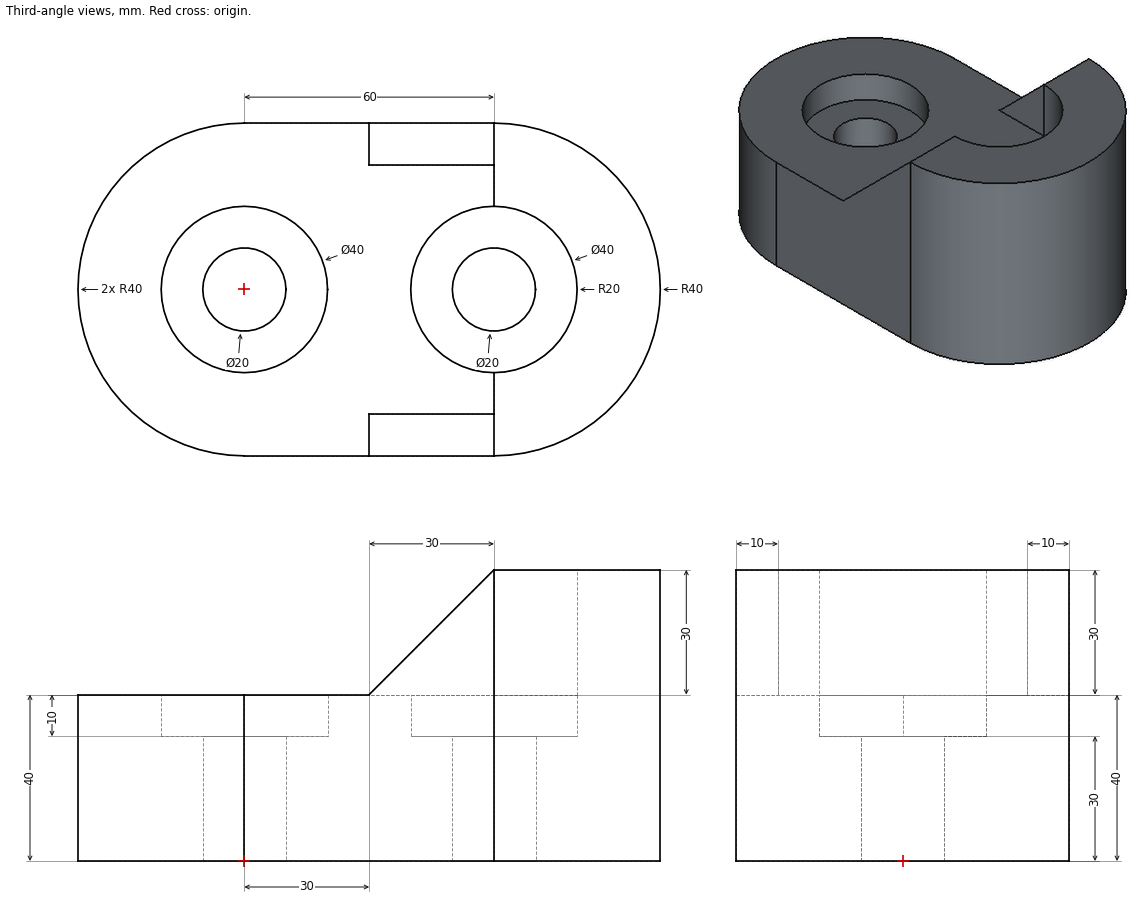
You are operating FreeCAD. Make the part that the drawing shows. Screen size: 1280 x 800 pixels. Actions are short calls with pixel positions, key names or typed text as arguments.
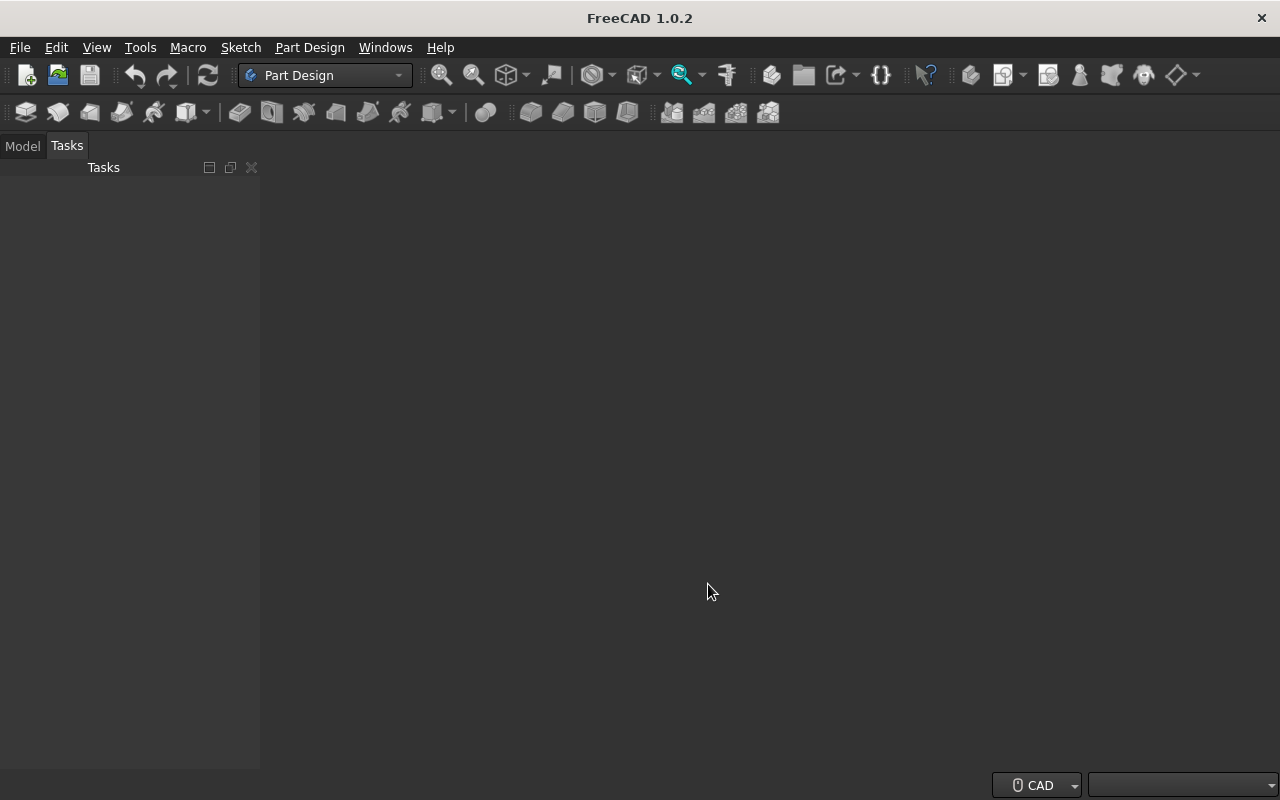
click(26, 76)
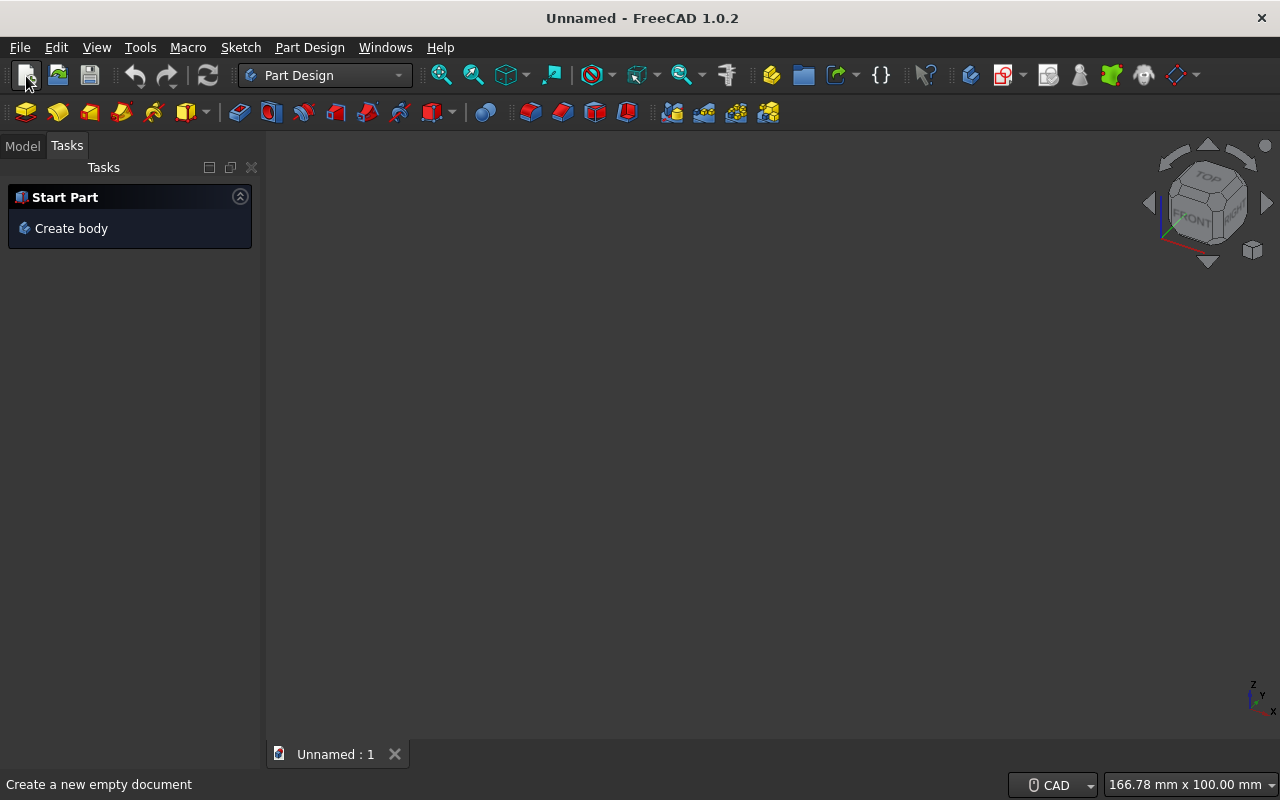
click(1004, 76)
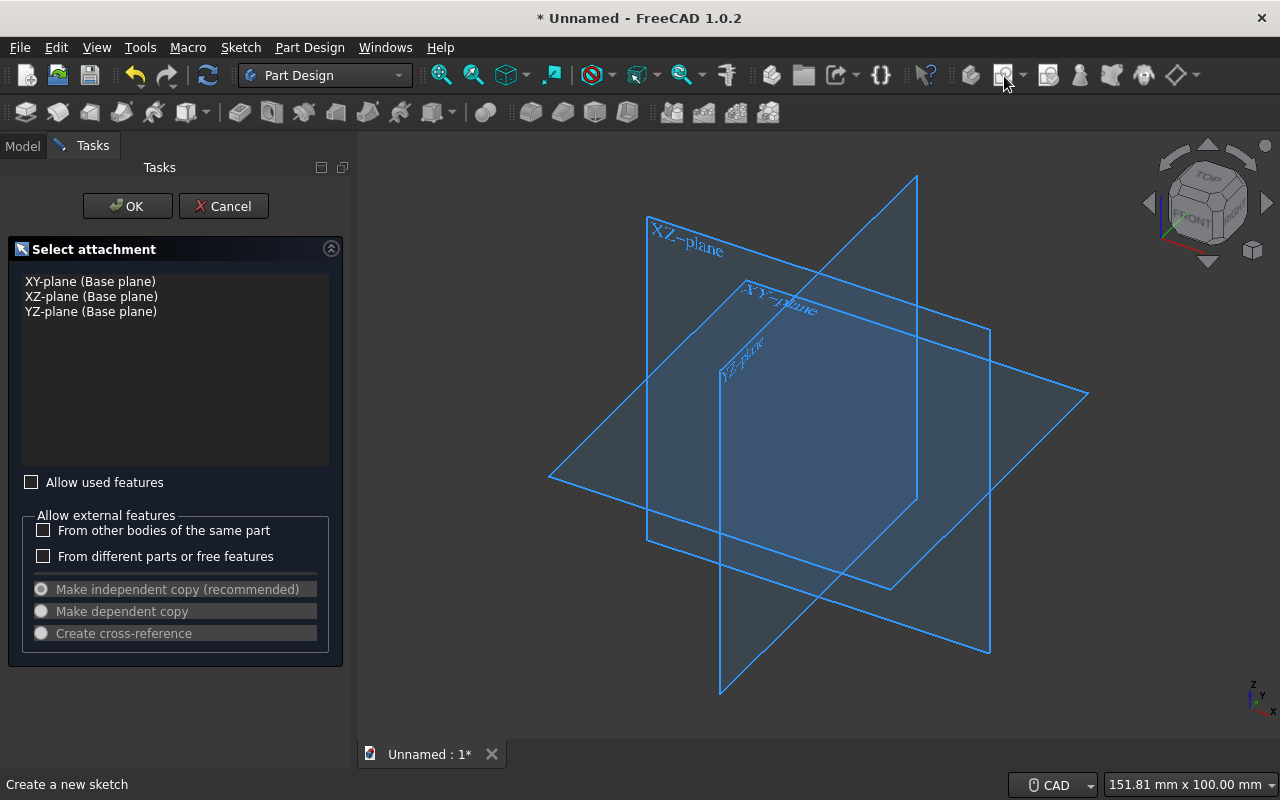
click(82, 282)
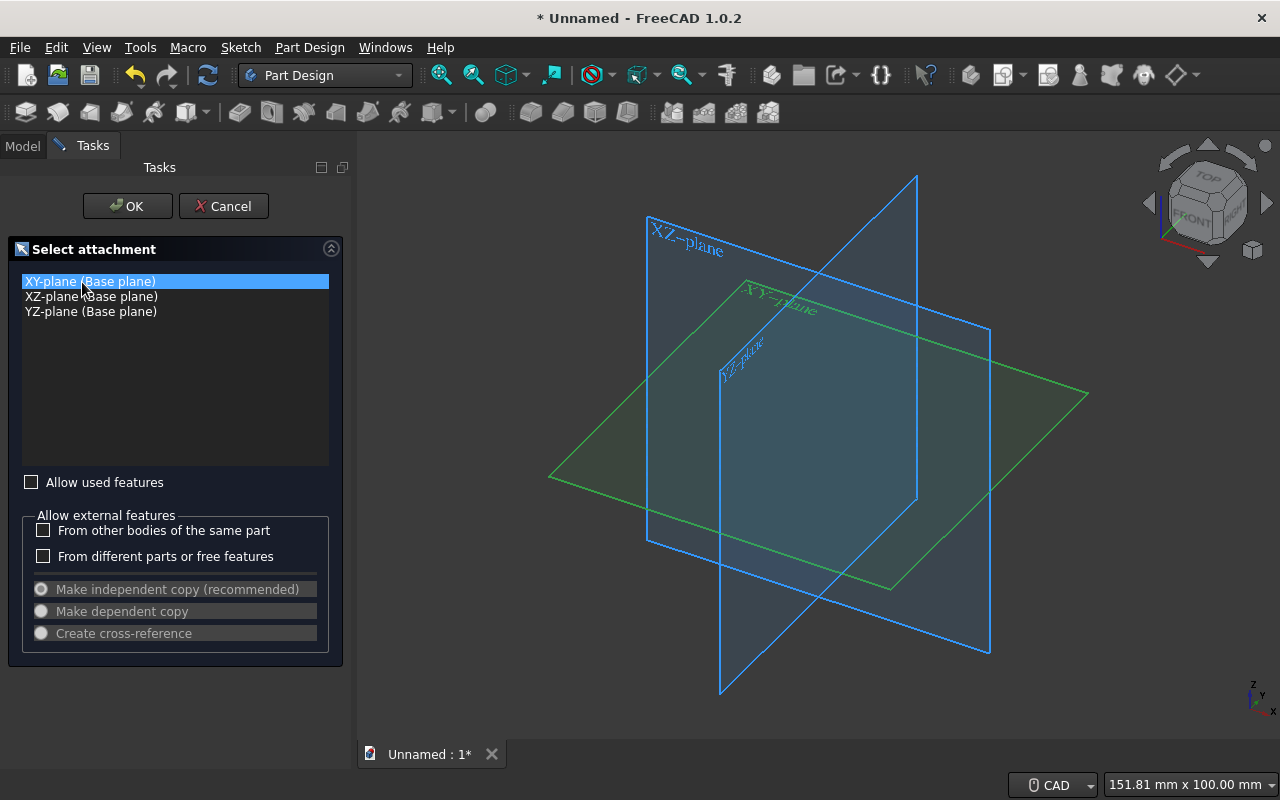
click(128, 206)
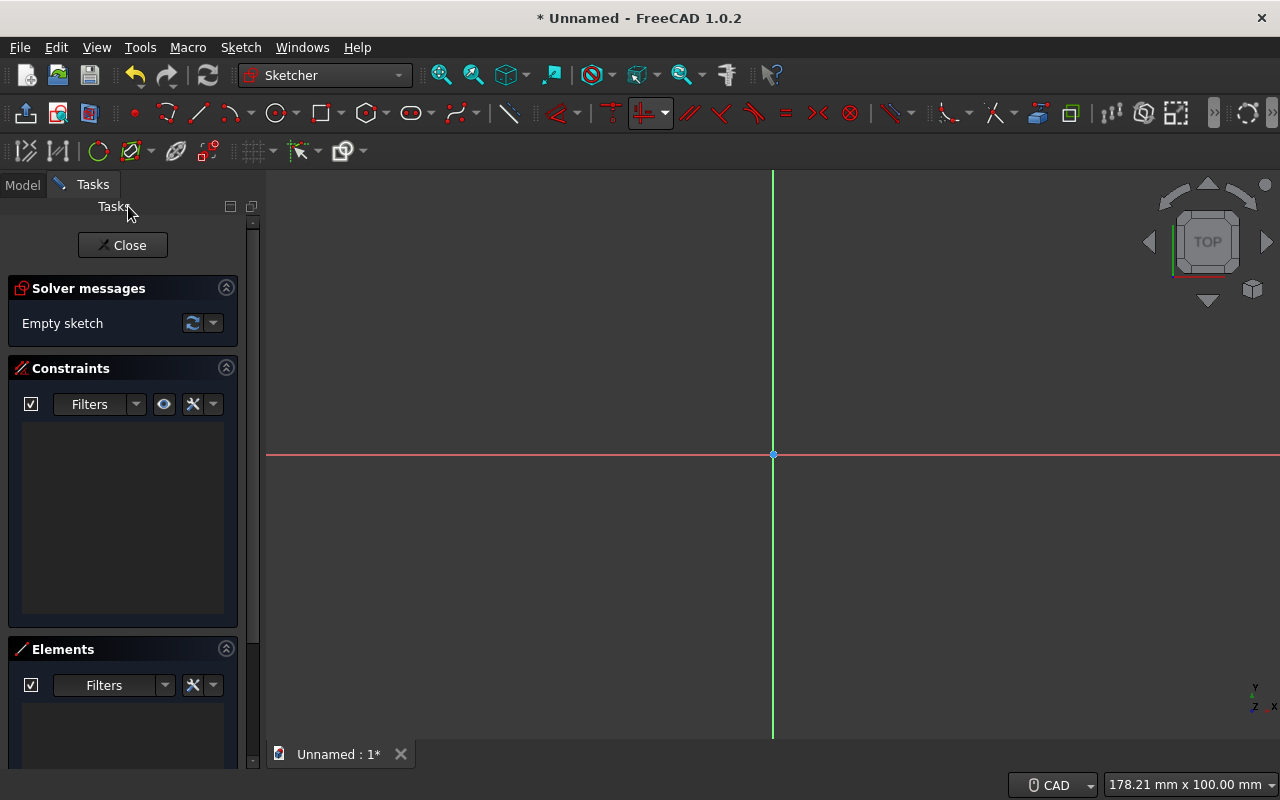
scroll(294, 455, down, 2)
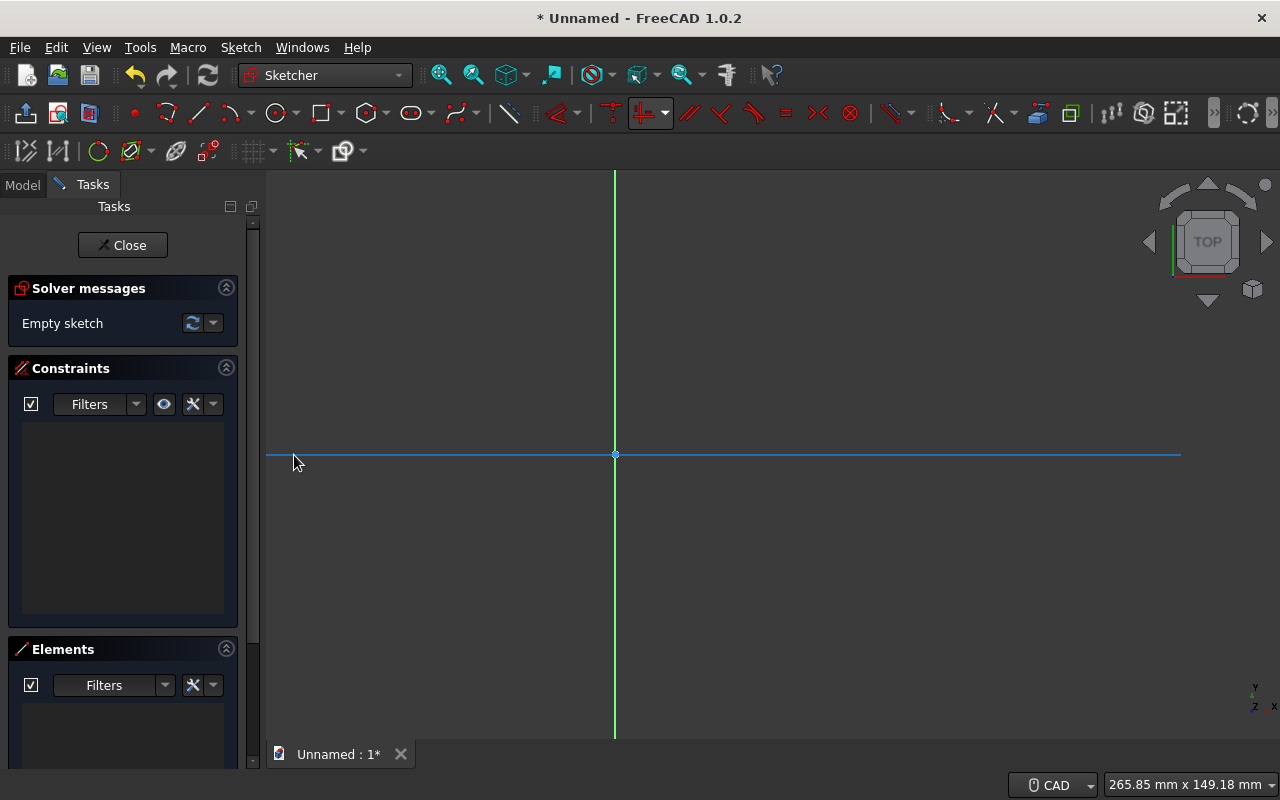
click(412, 114)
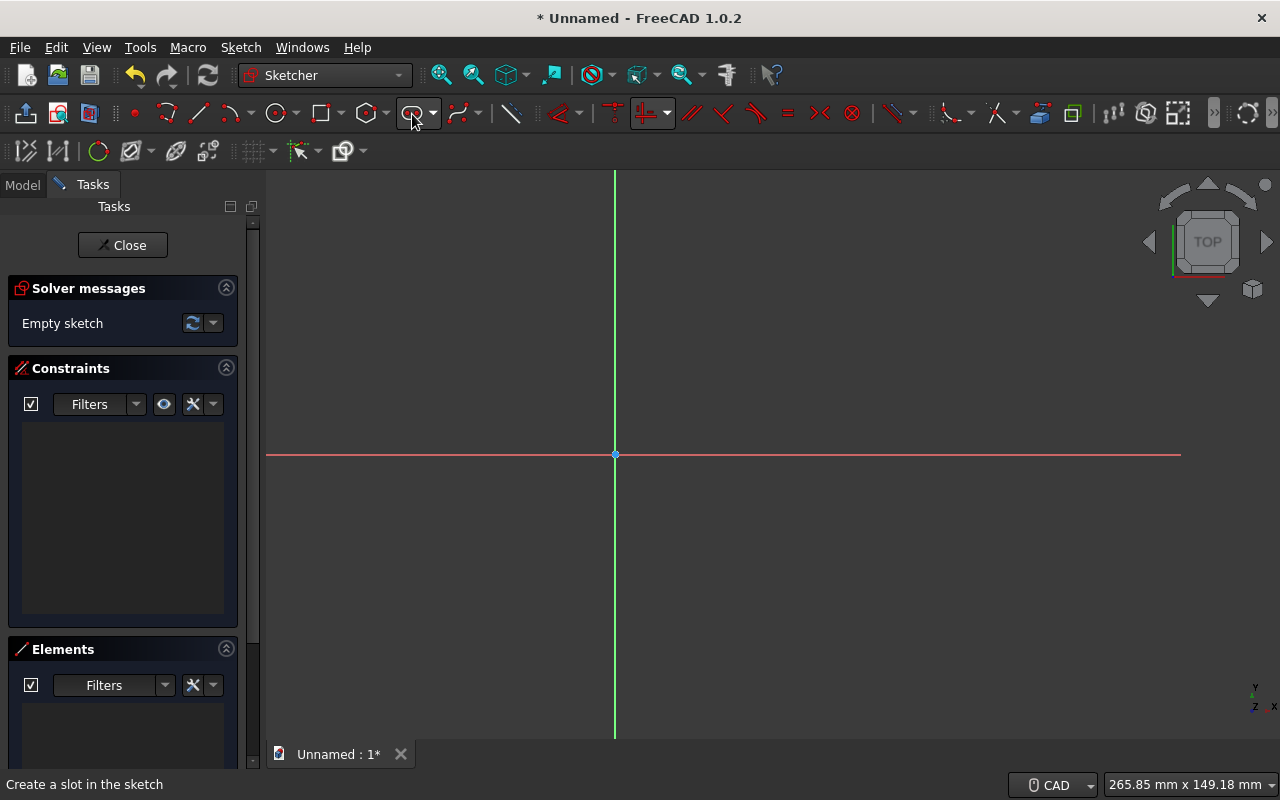
click(615, 455)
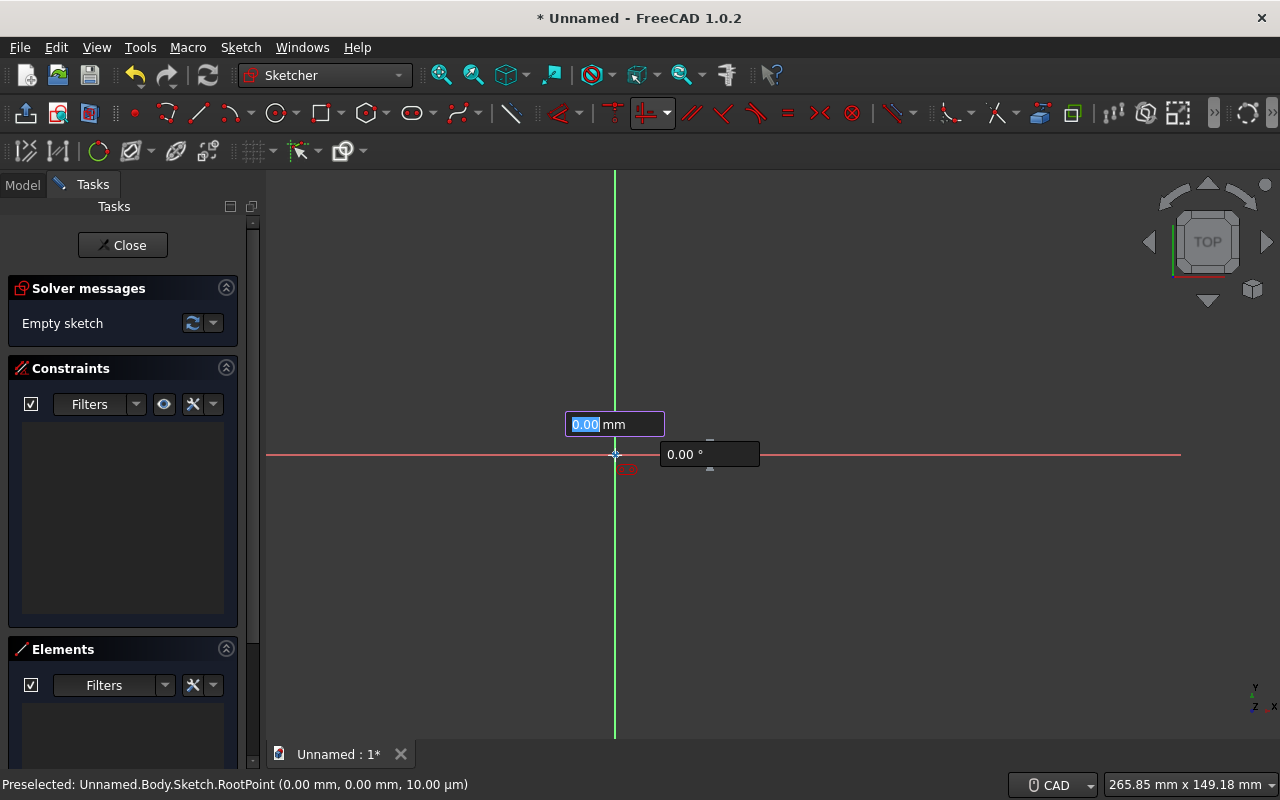
click(844, 446)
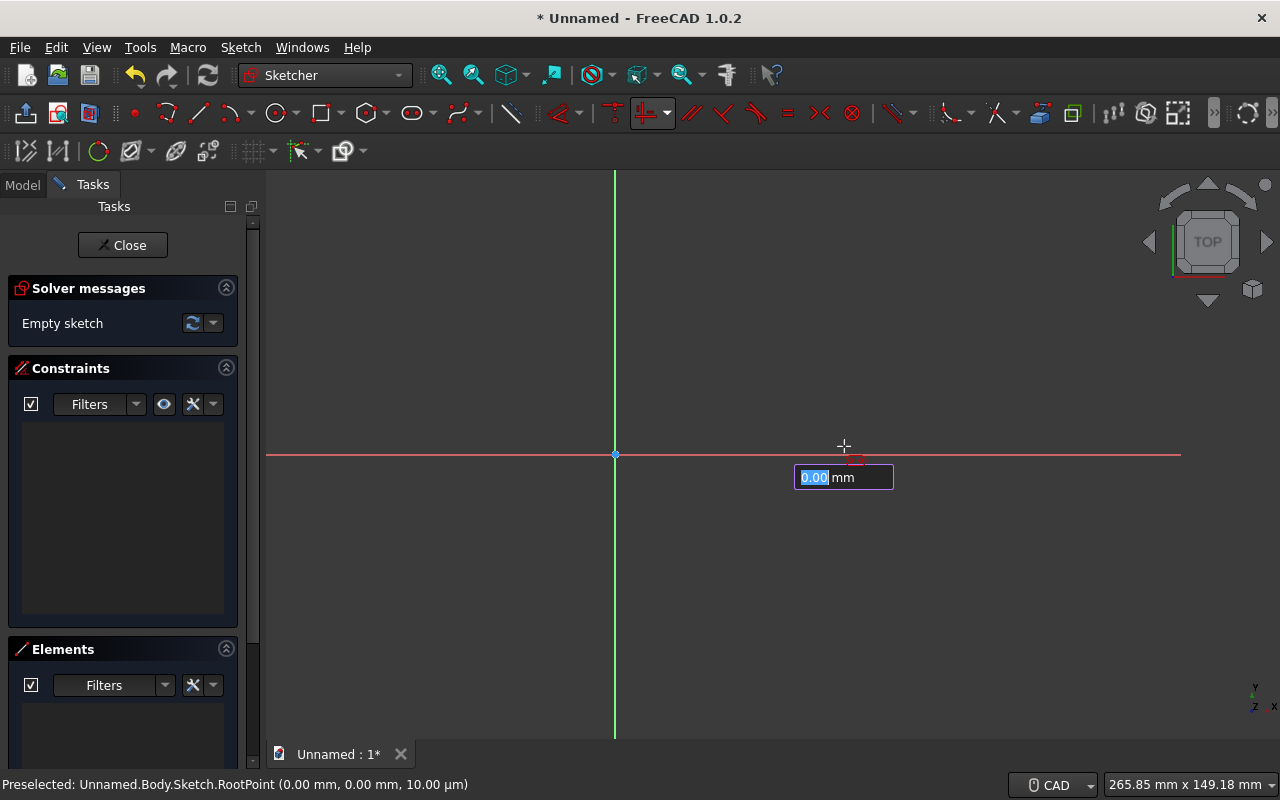
click(730, 302)
key(Escape)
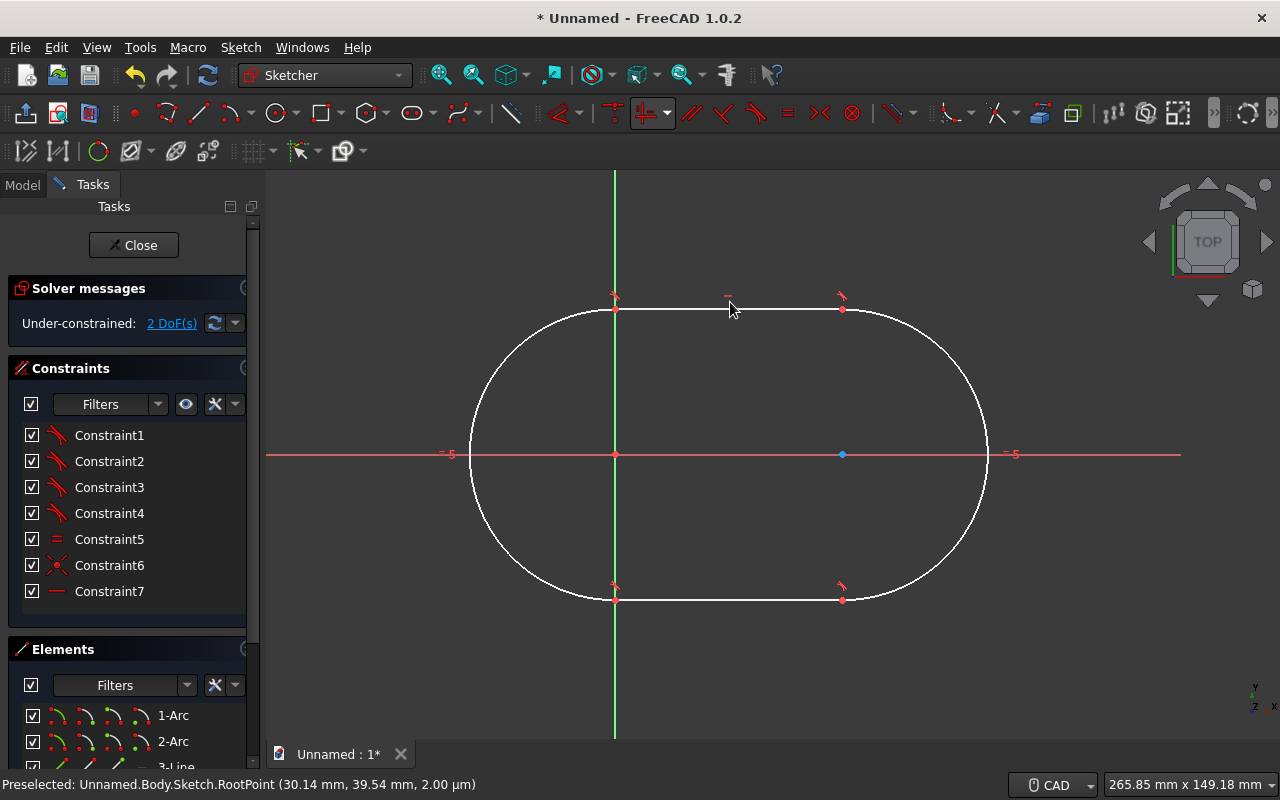
click(558, 114)